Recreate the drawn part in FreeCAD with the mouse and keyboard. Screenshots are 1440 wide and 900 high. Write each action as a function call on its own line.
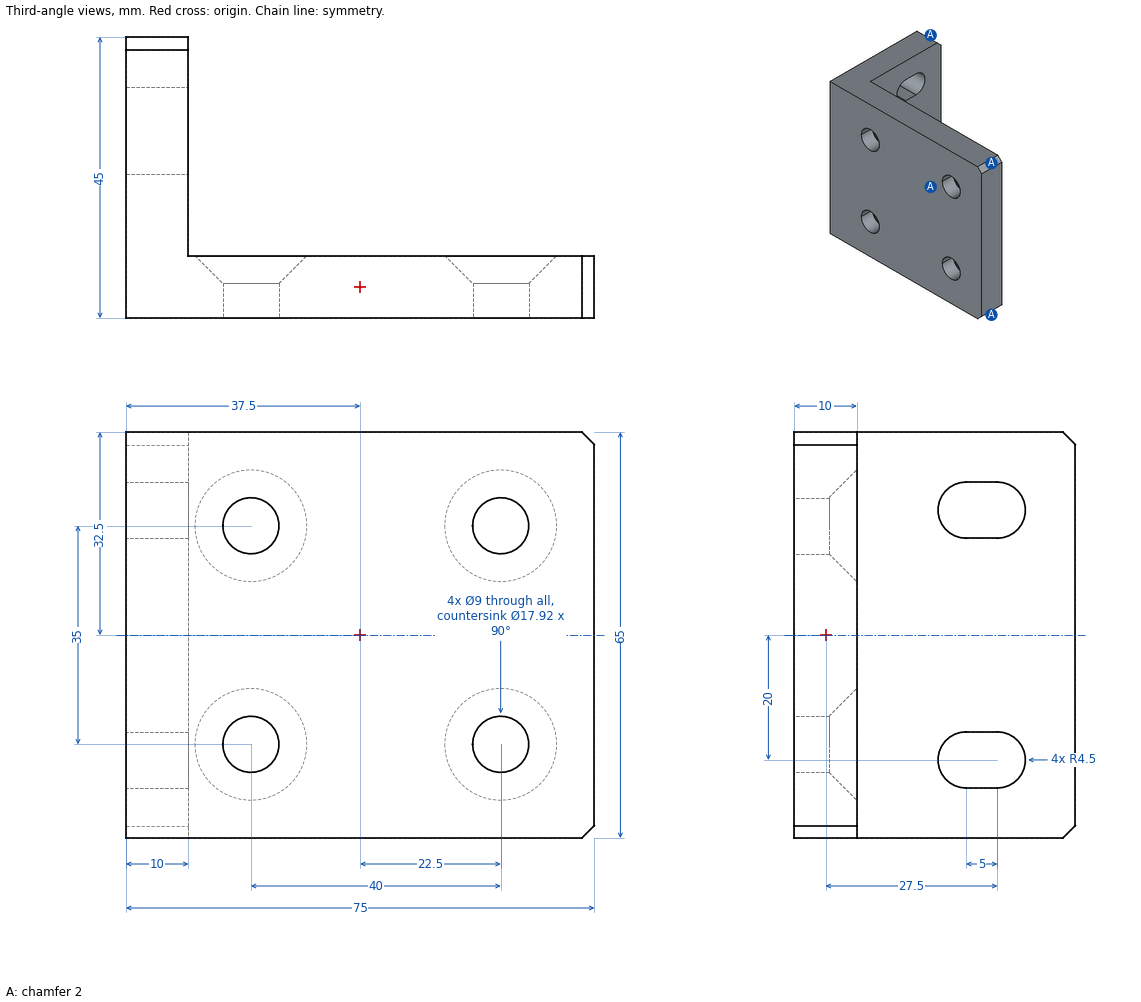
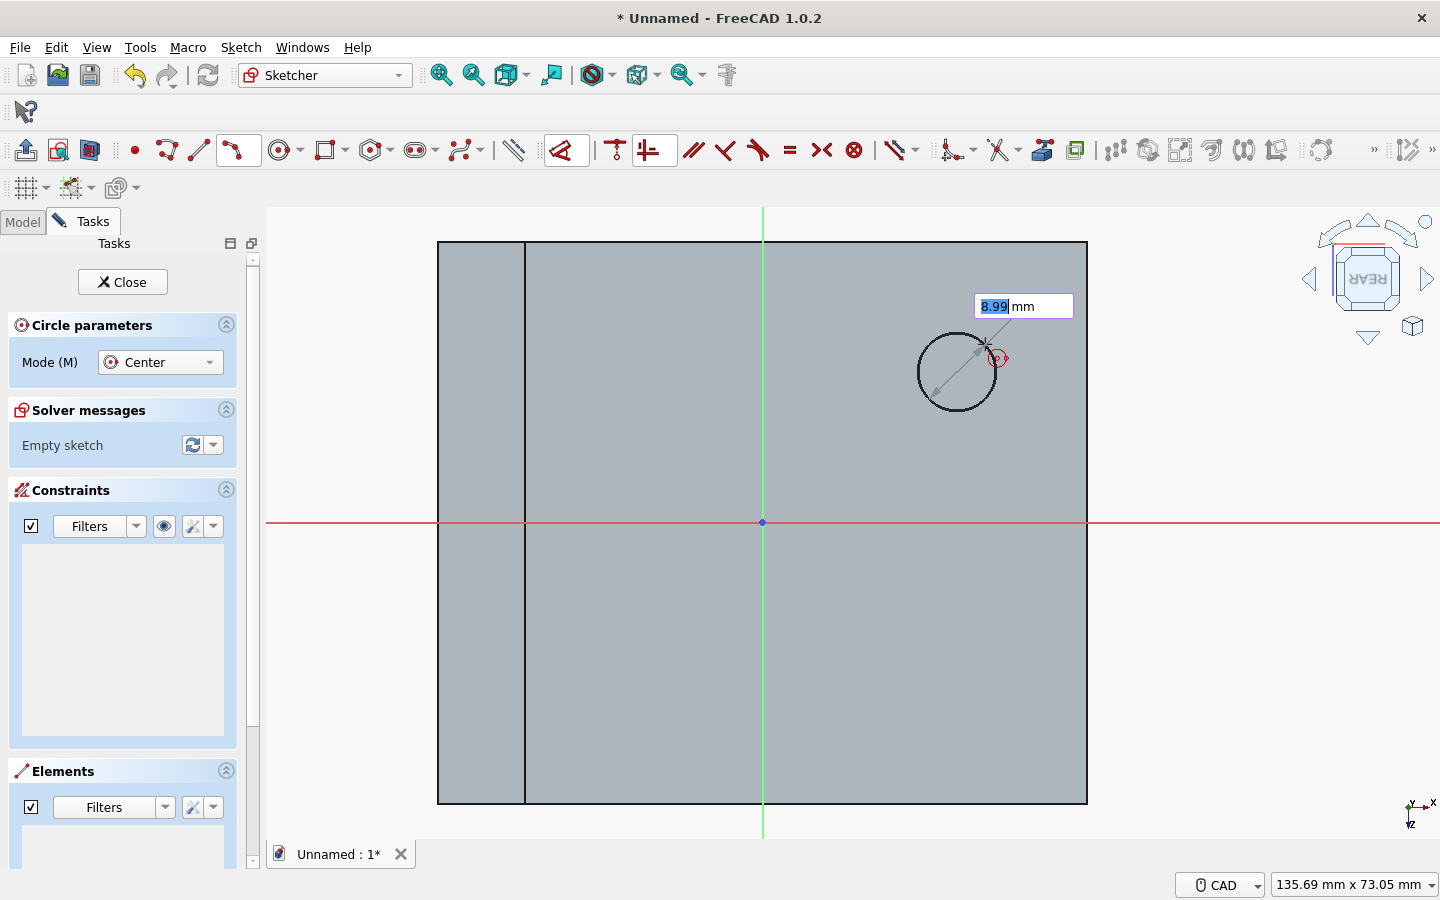
text(9)
key(Return)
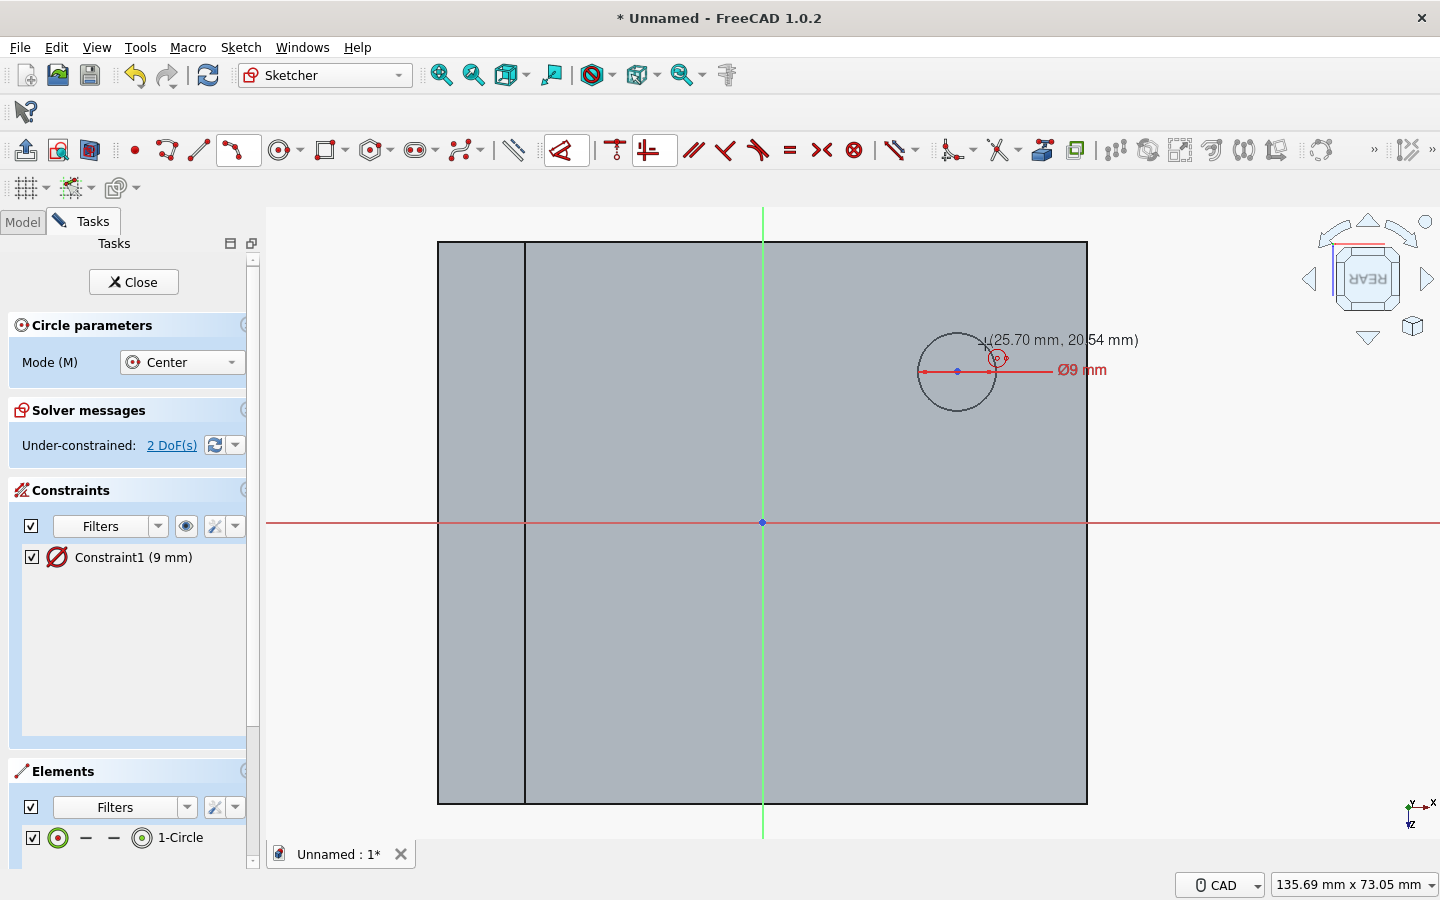
click(611, 371)
move(639, 344)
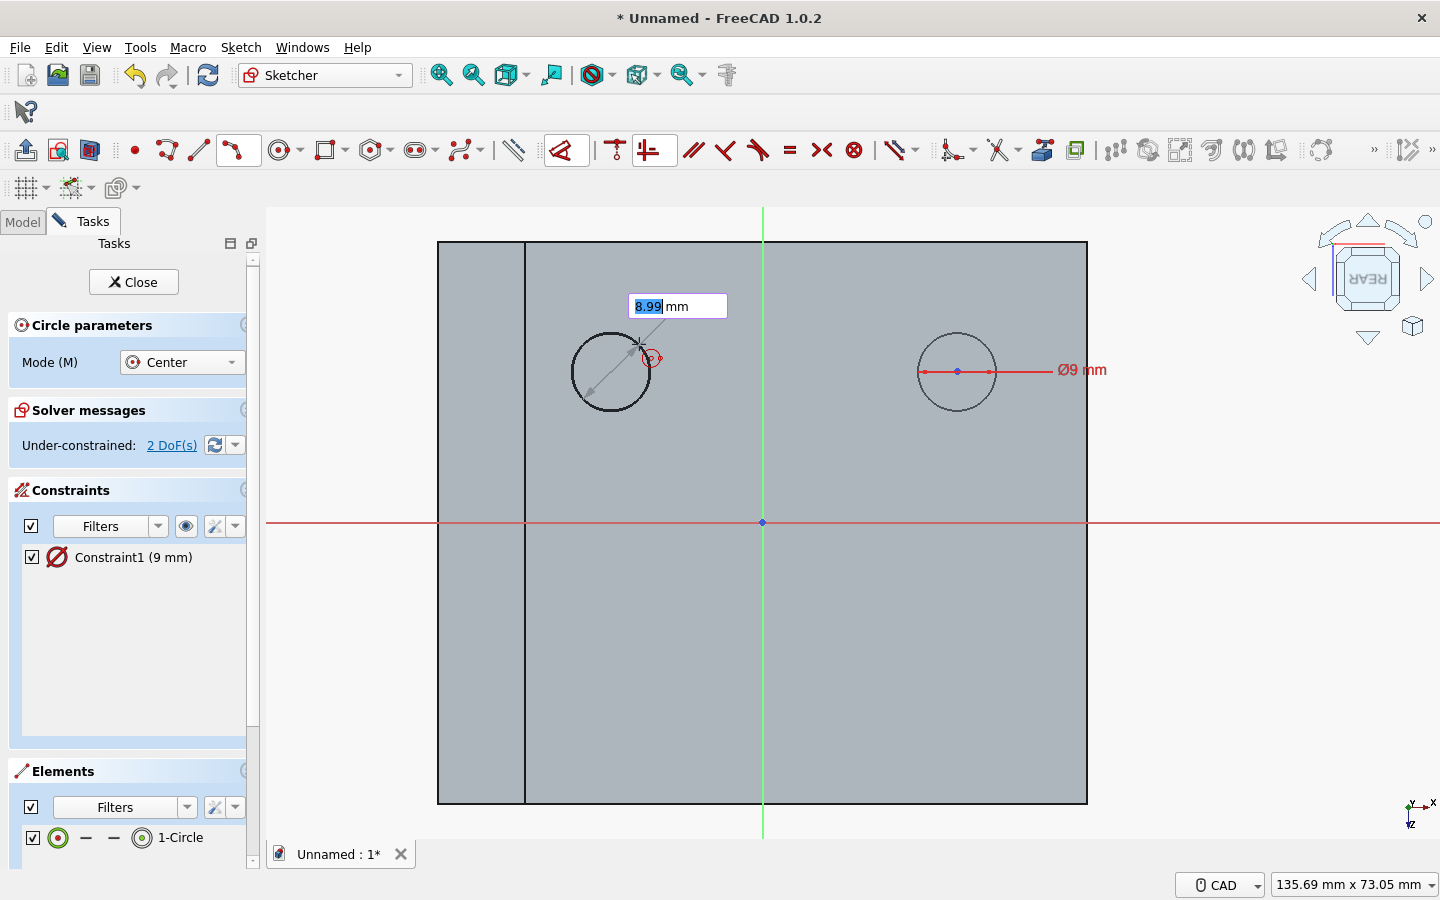
text(9)
key(Return)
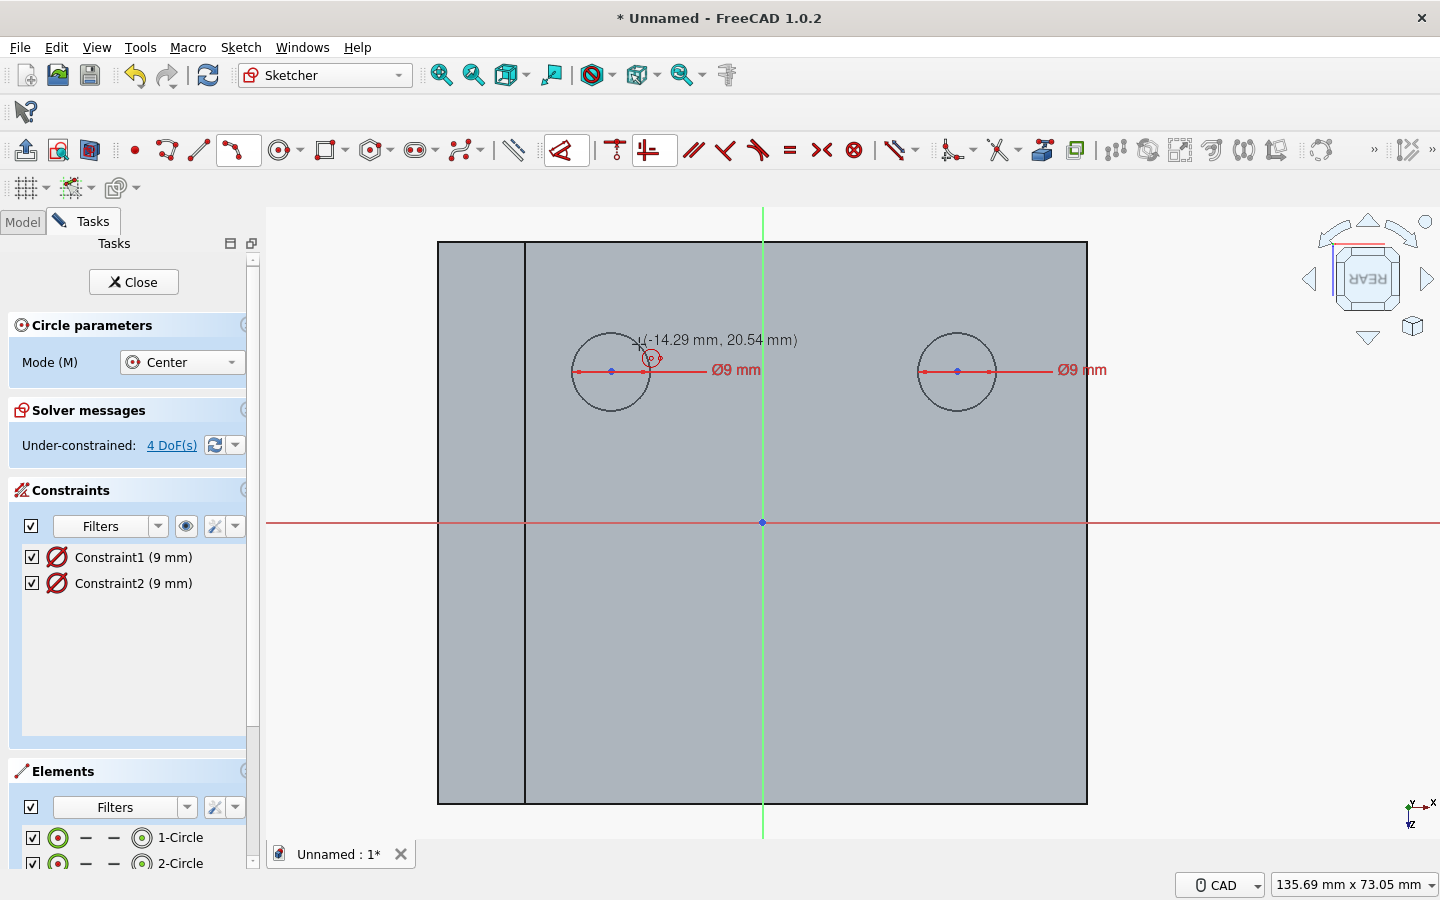
click(611, 674)
move(639, 647)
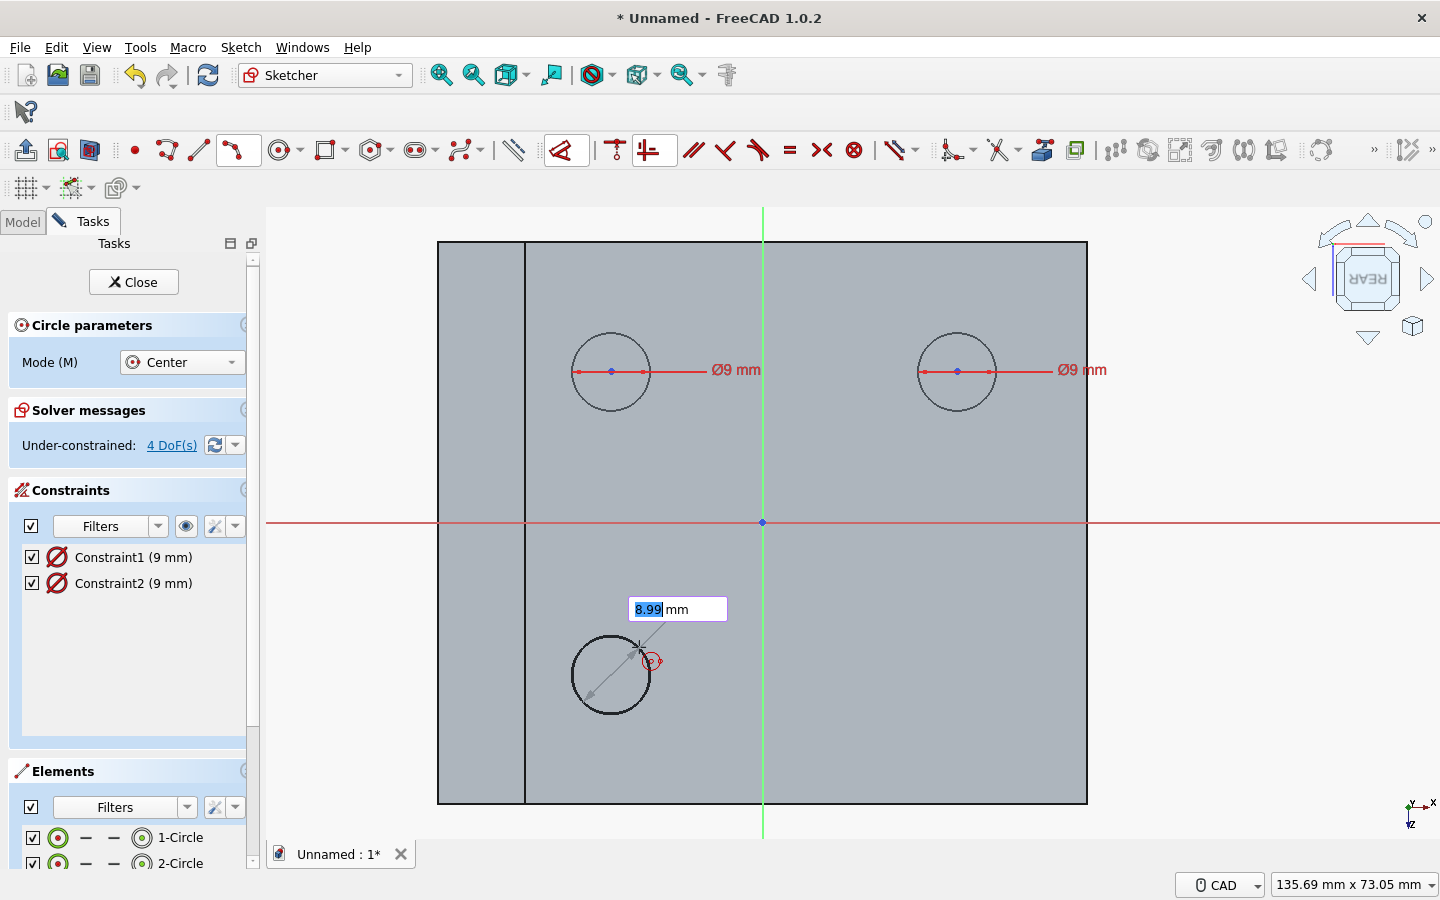
text(9)
key(Return)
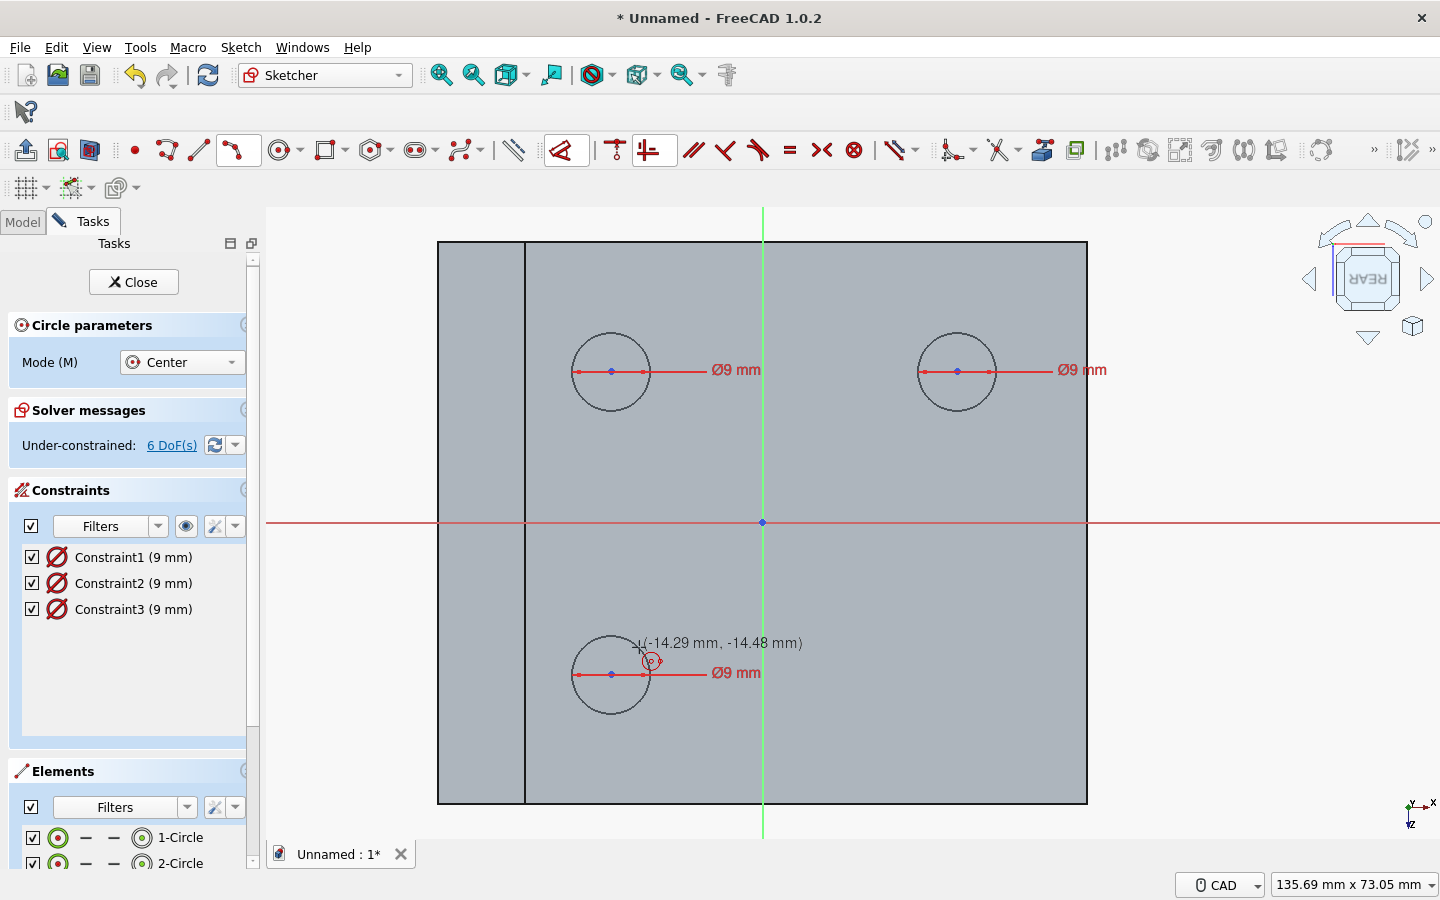
click(957, 674)
move(985, 647)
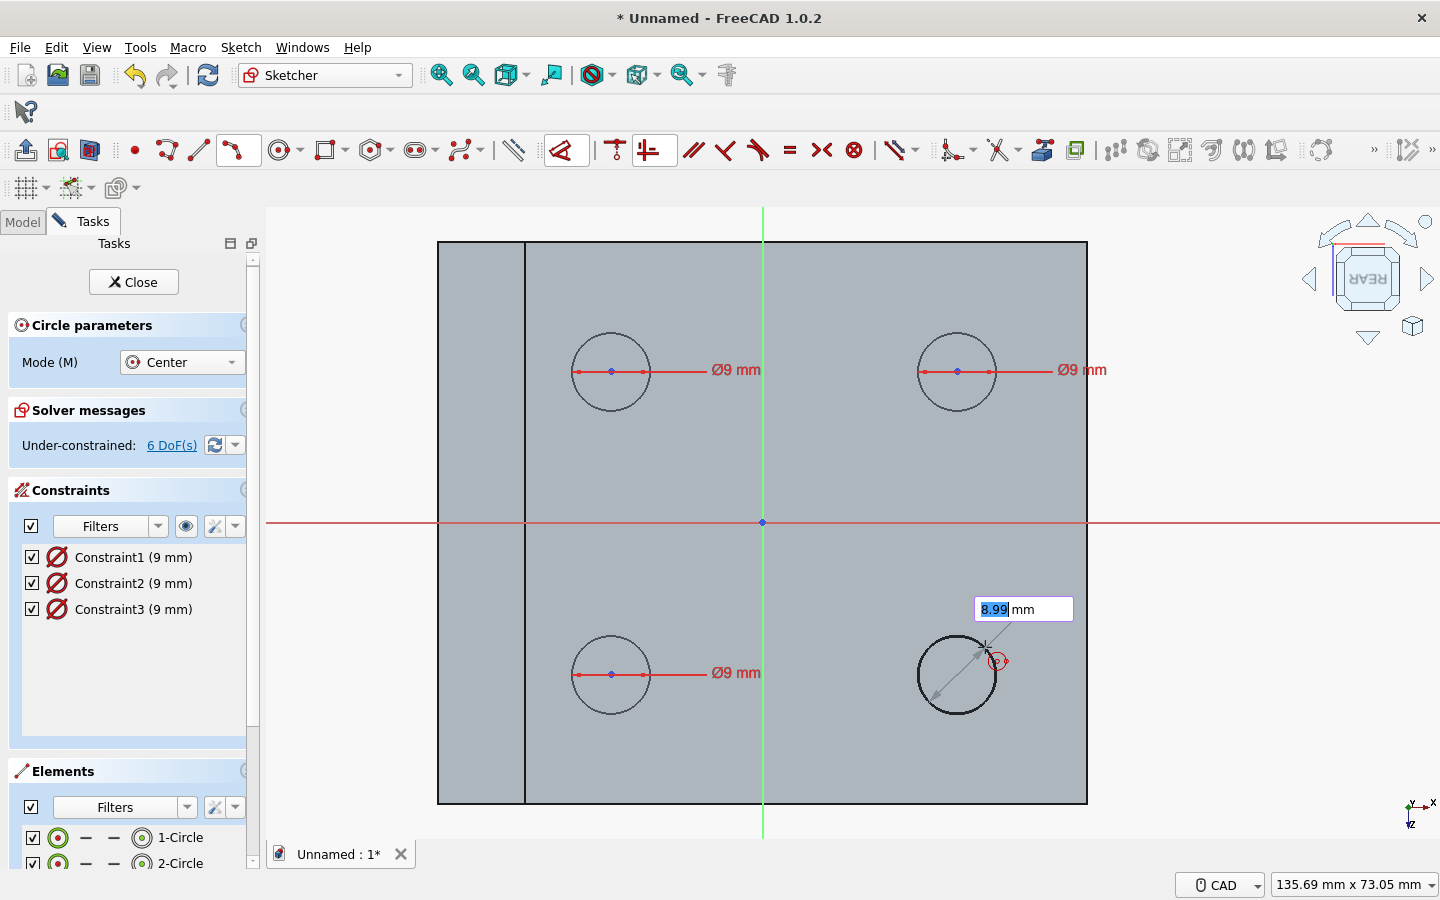
text(9)
key(Return)
key(Escape)